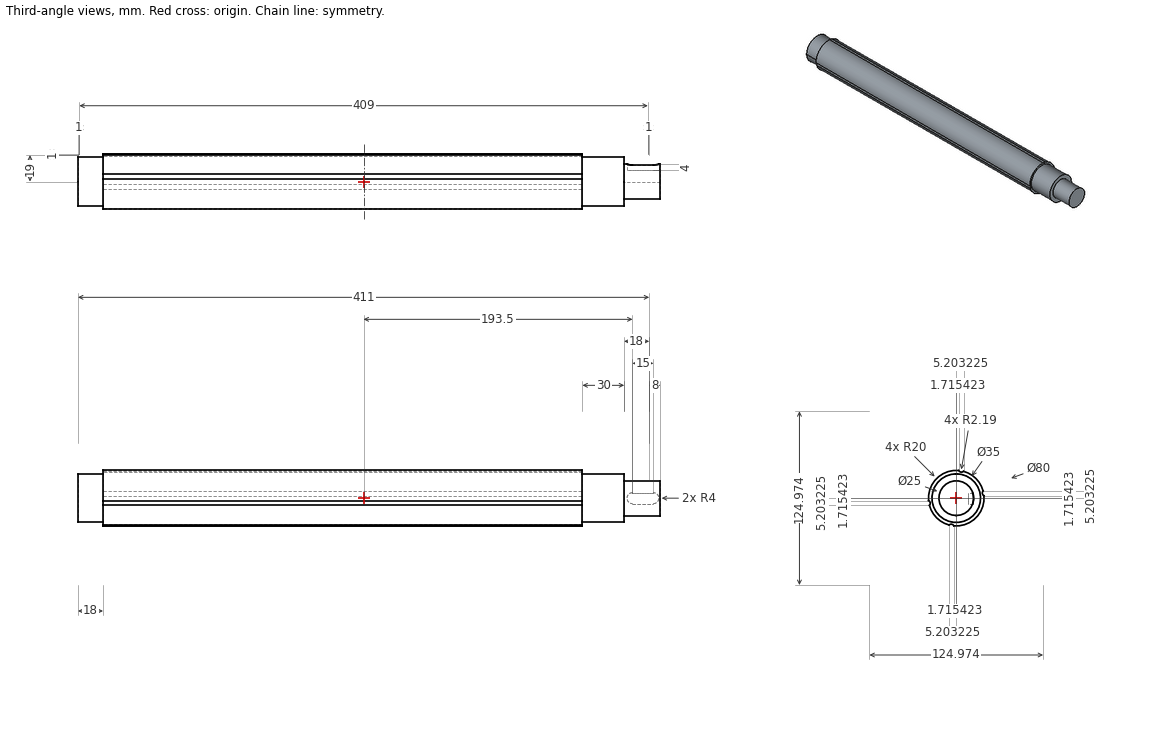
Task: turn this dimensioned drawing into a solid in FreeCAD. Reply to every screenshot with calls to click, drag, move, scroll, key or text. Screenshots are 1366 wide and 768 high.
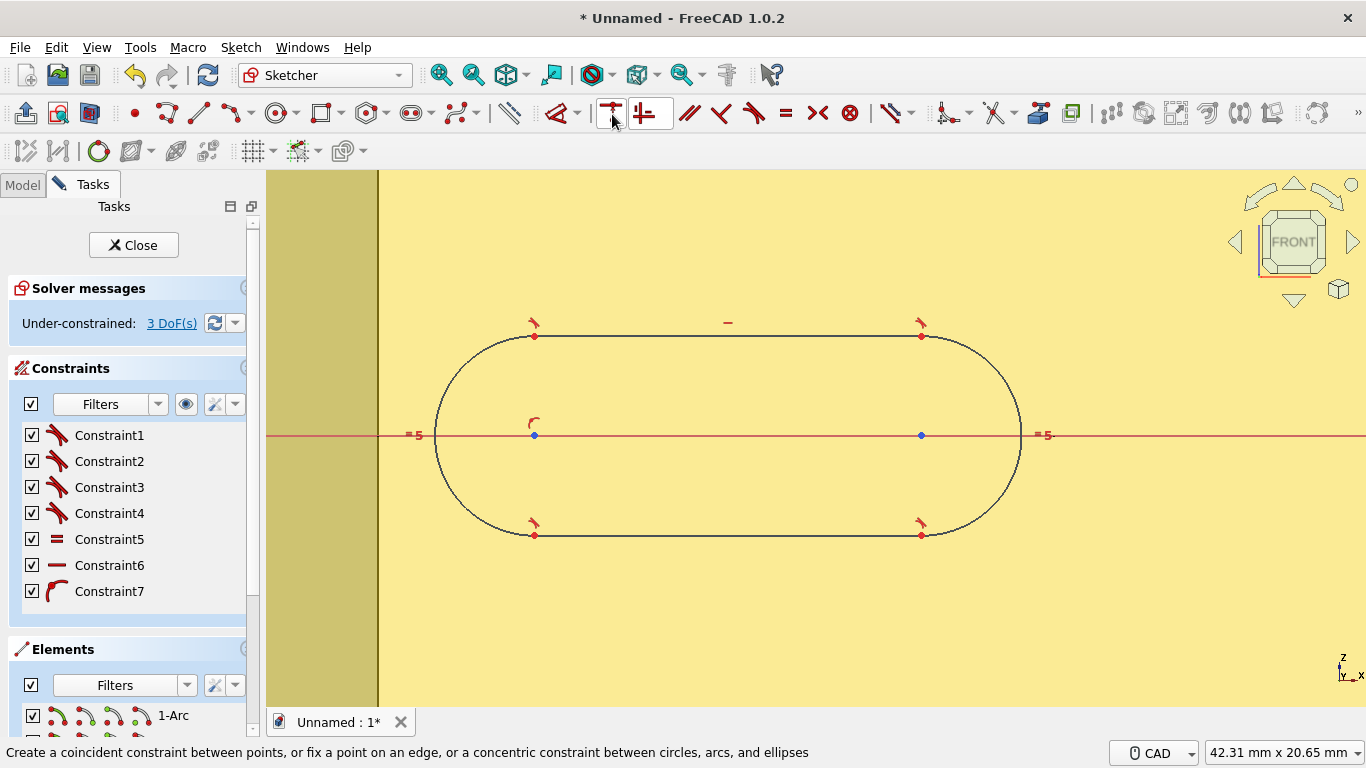
click(454, 377)
click(428, 358)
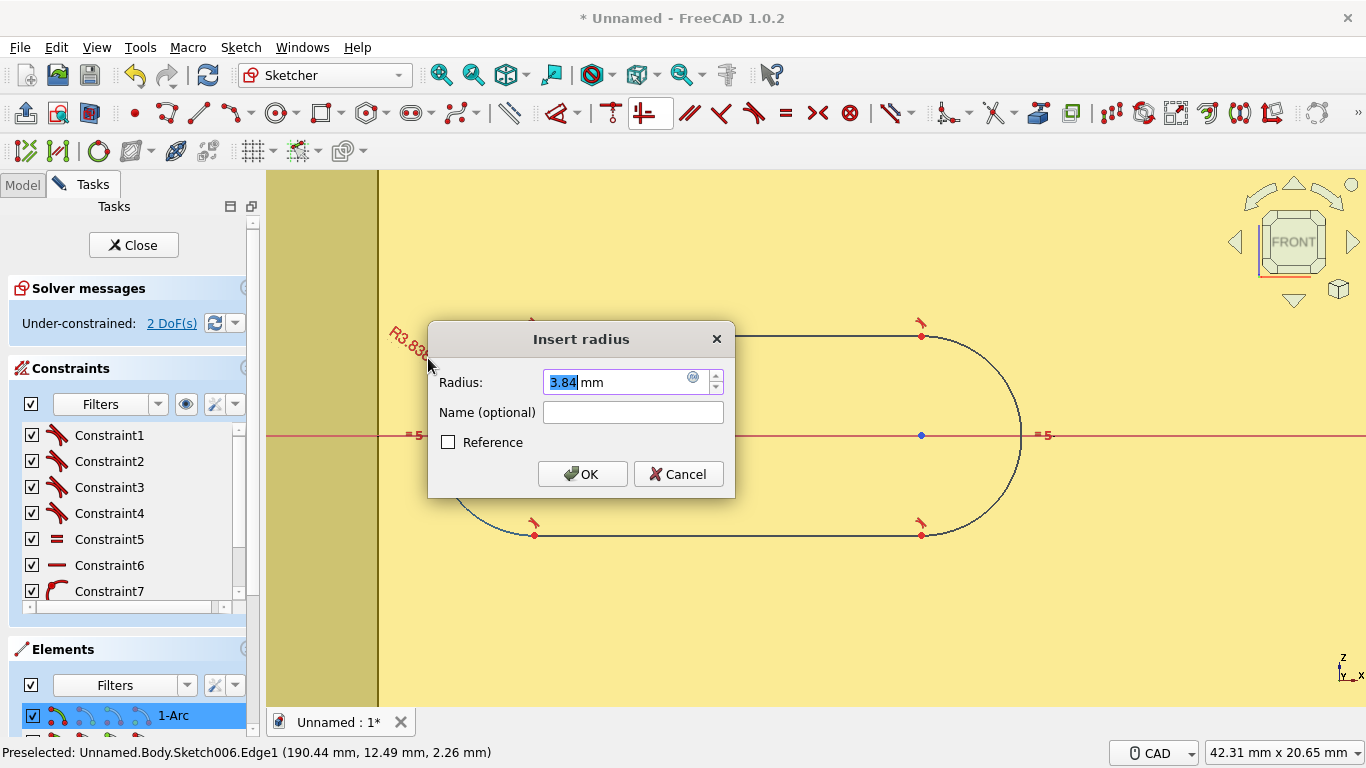
text(4)
key(Return)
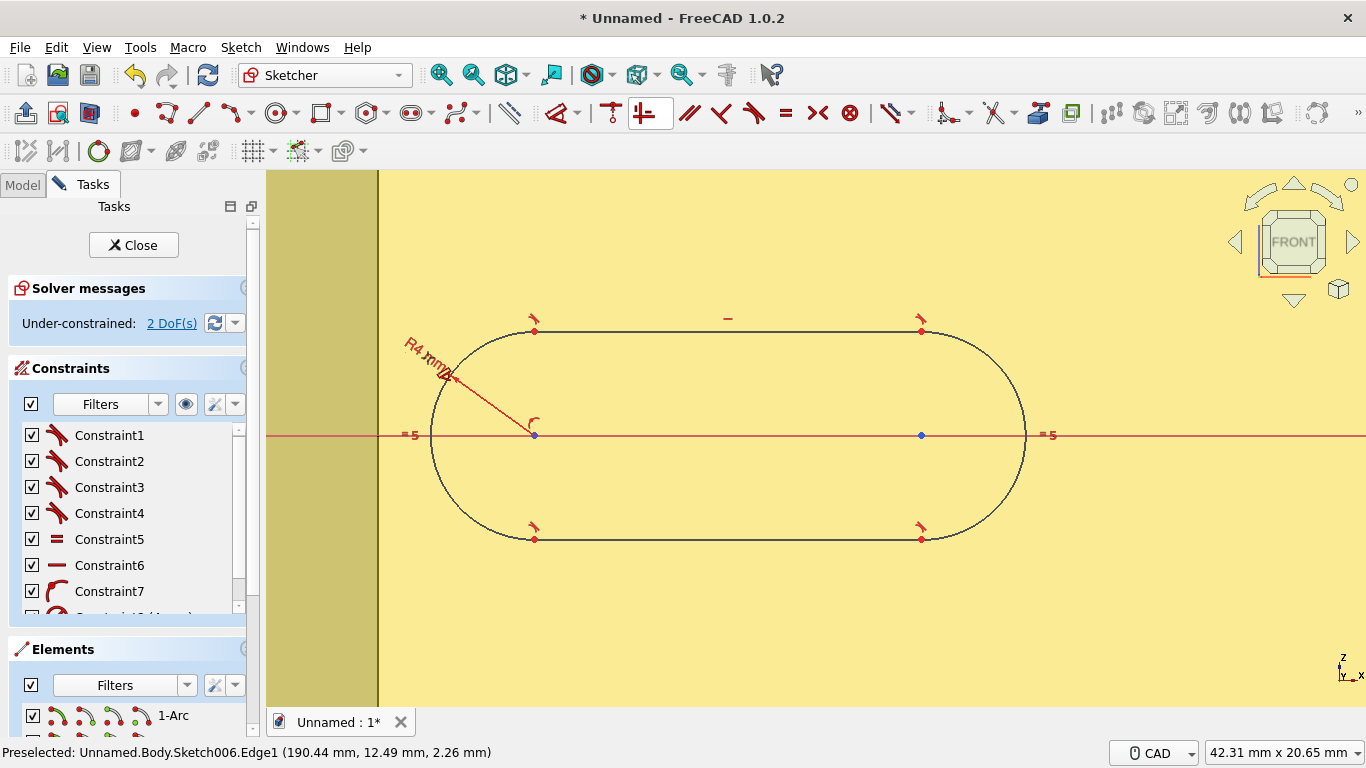
click(651, 332)
click(728, 298)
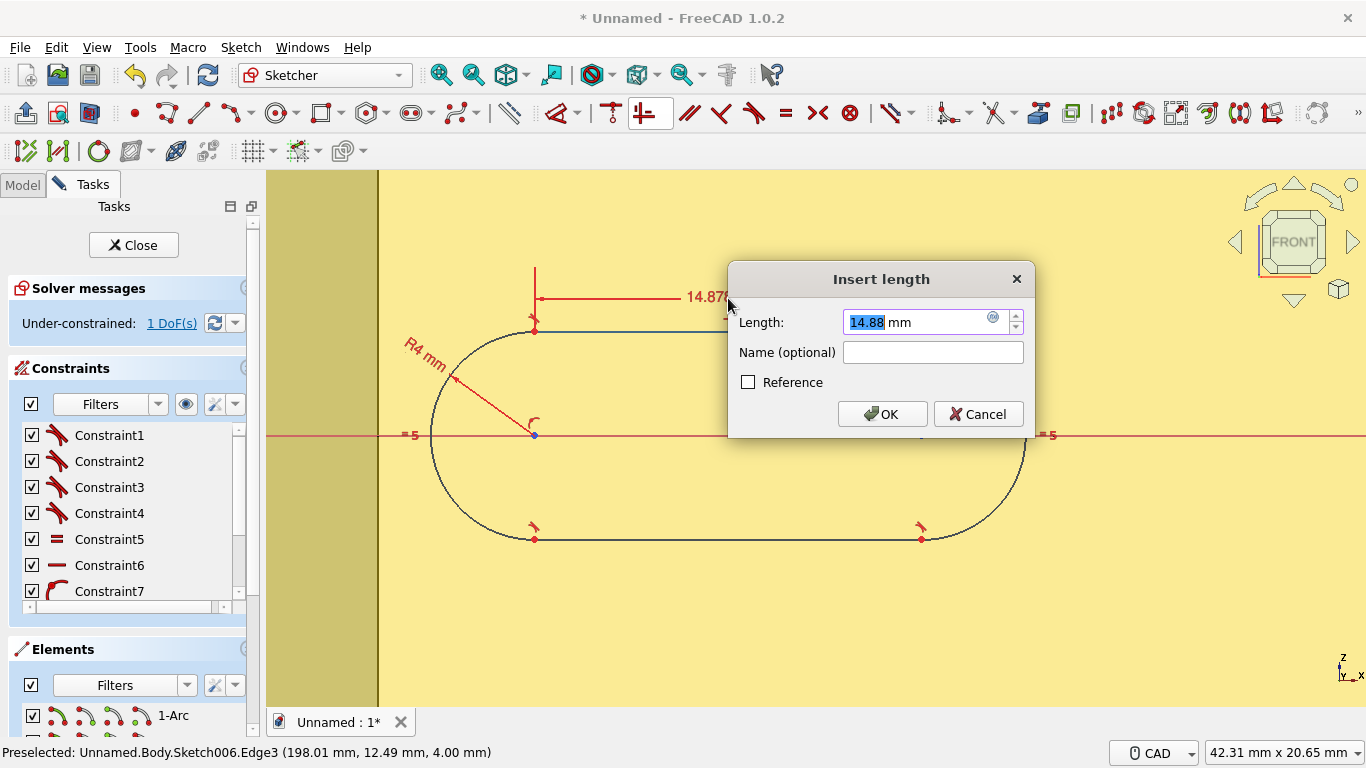
text(15)
key(Return)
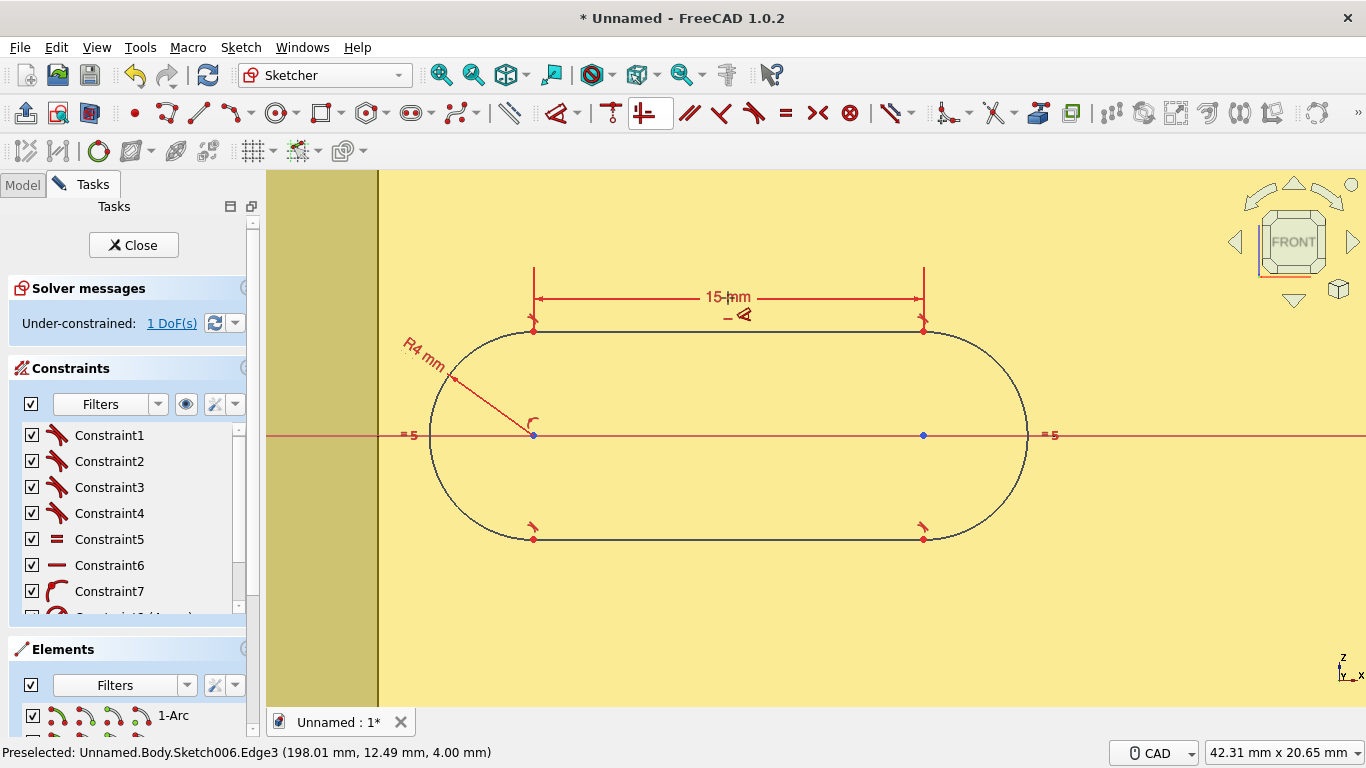
click(534, 332)
click(414, 298)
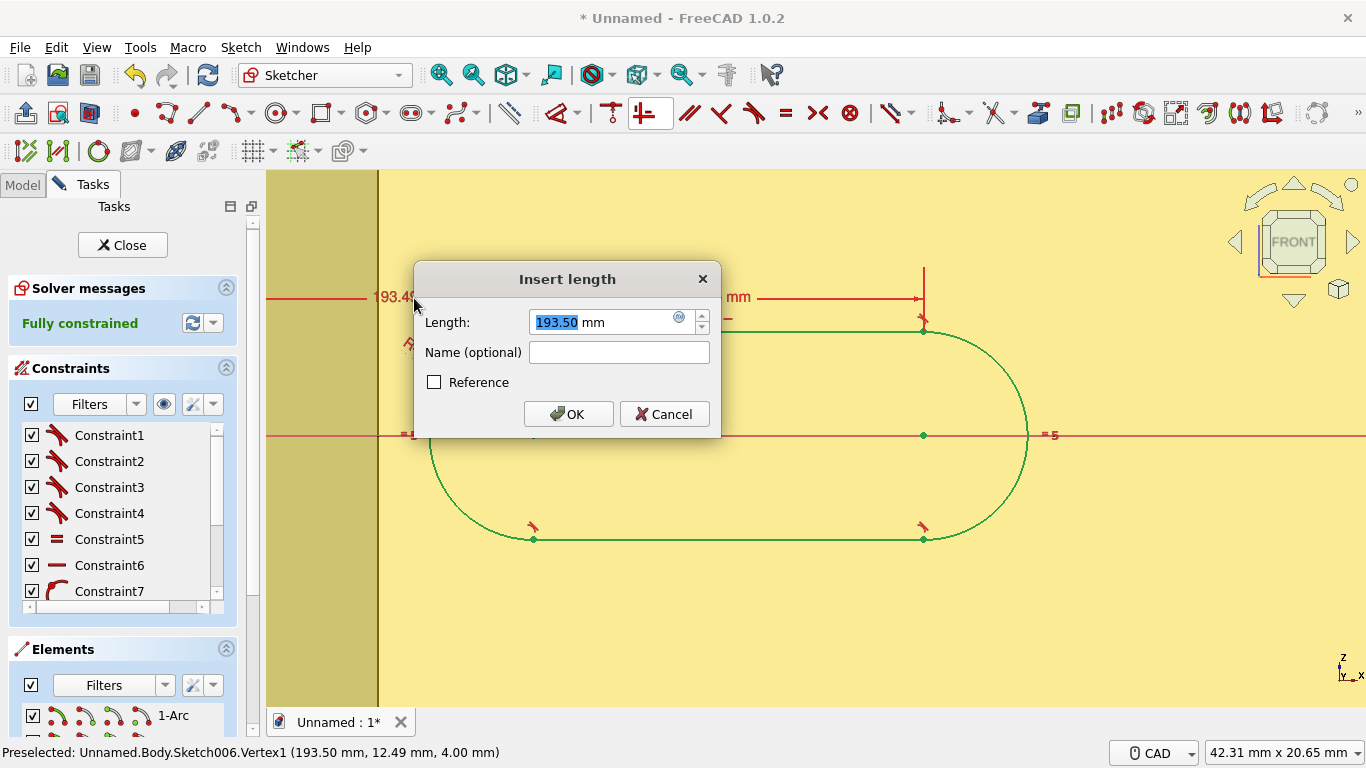
text(193.5)
key(Return)
key(Escape)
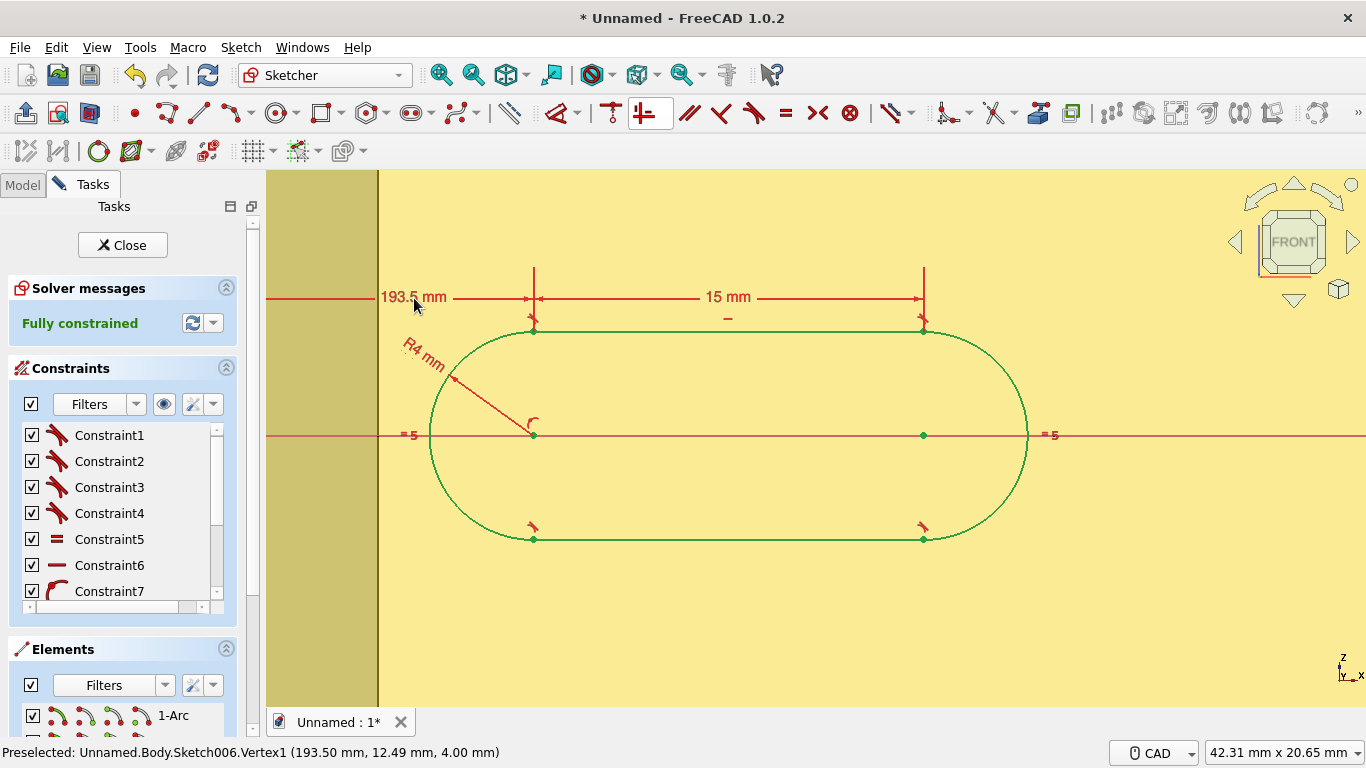
click(123, 245)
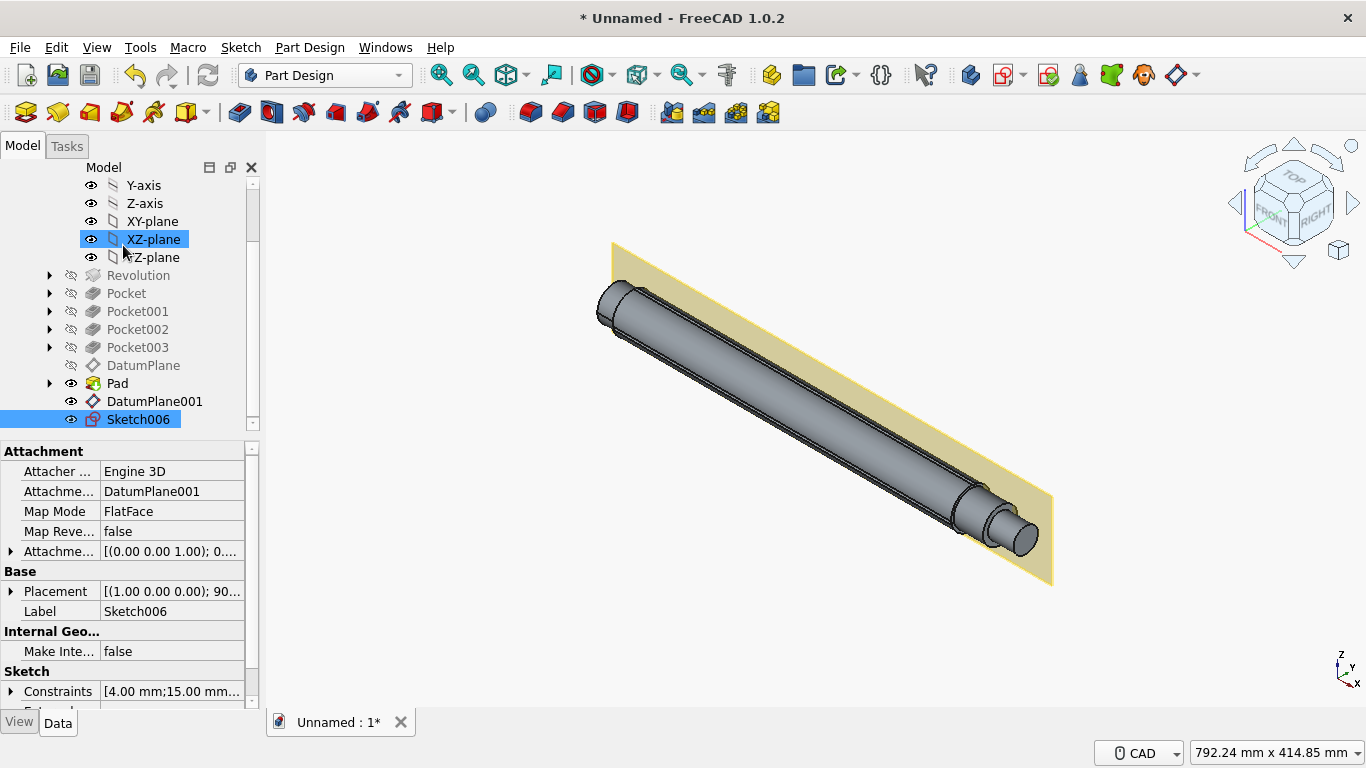
click(240, 112)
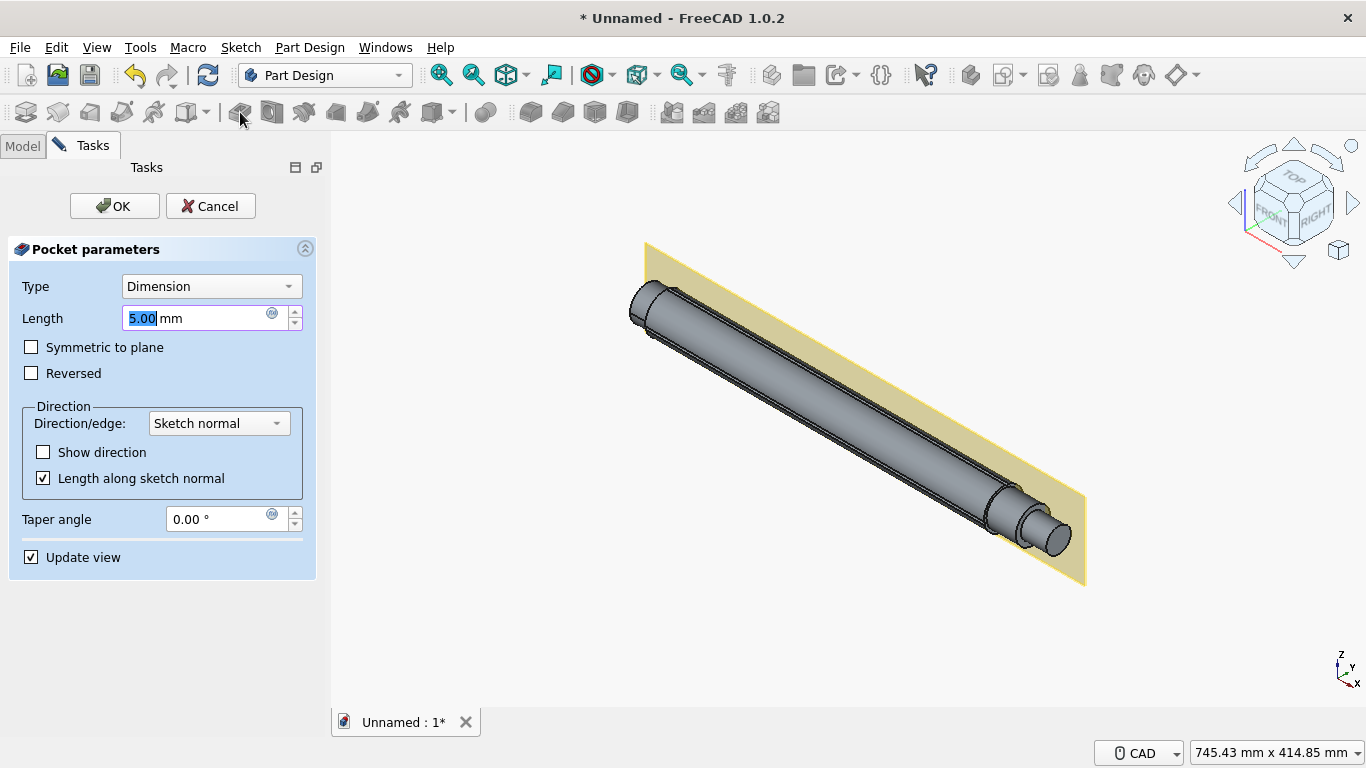
text(4)
key(Tab)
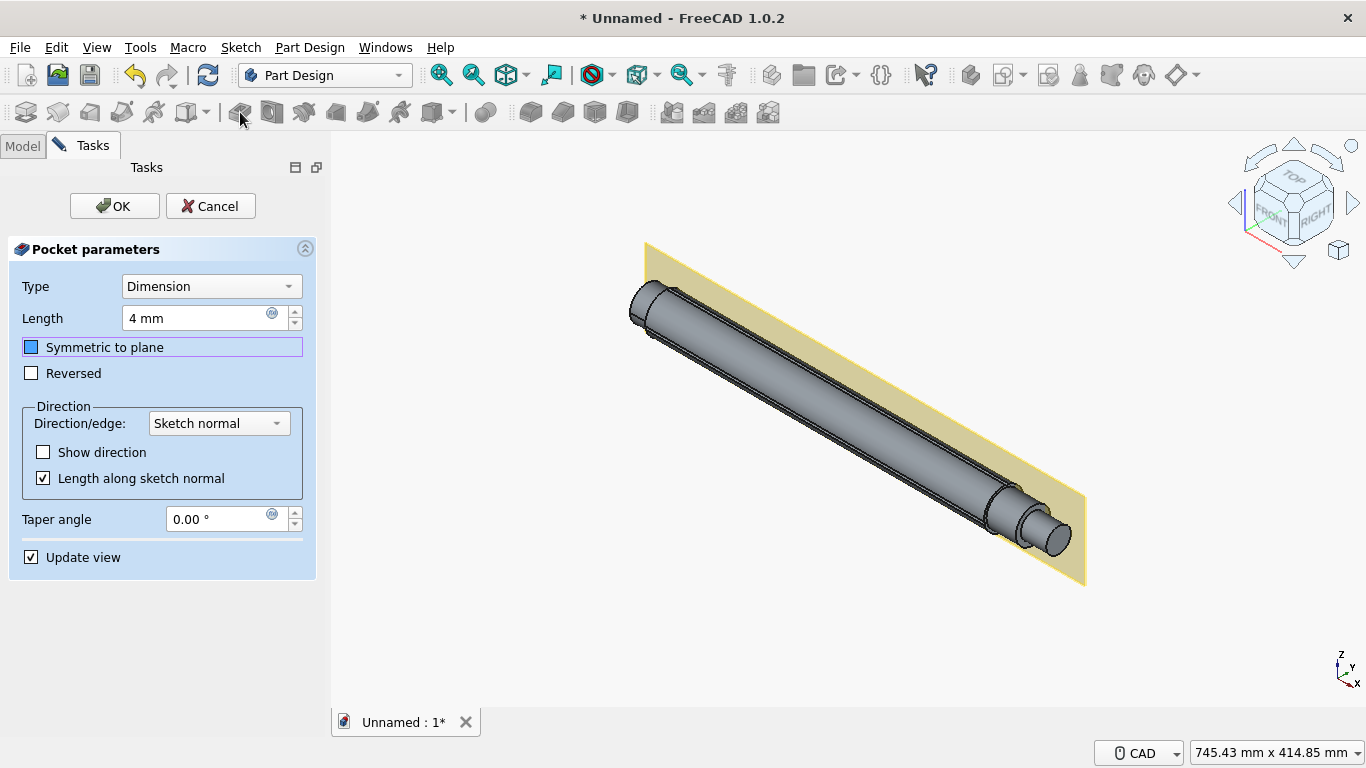
click(30, 373)